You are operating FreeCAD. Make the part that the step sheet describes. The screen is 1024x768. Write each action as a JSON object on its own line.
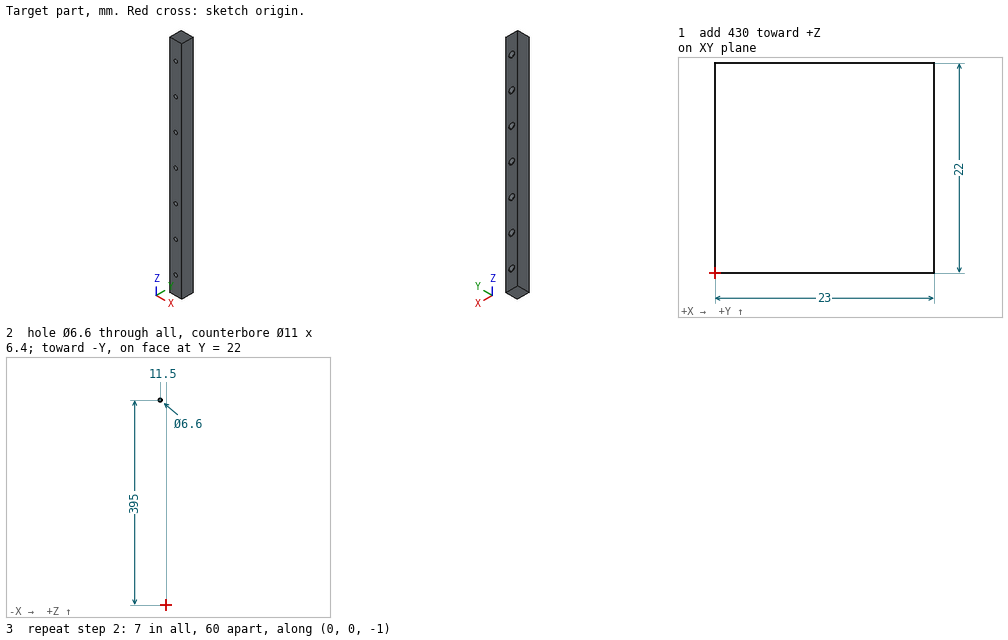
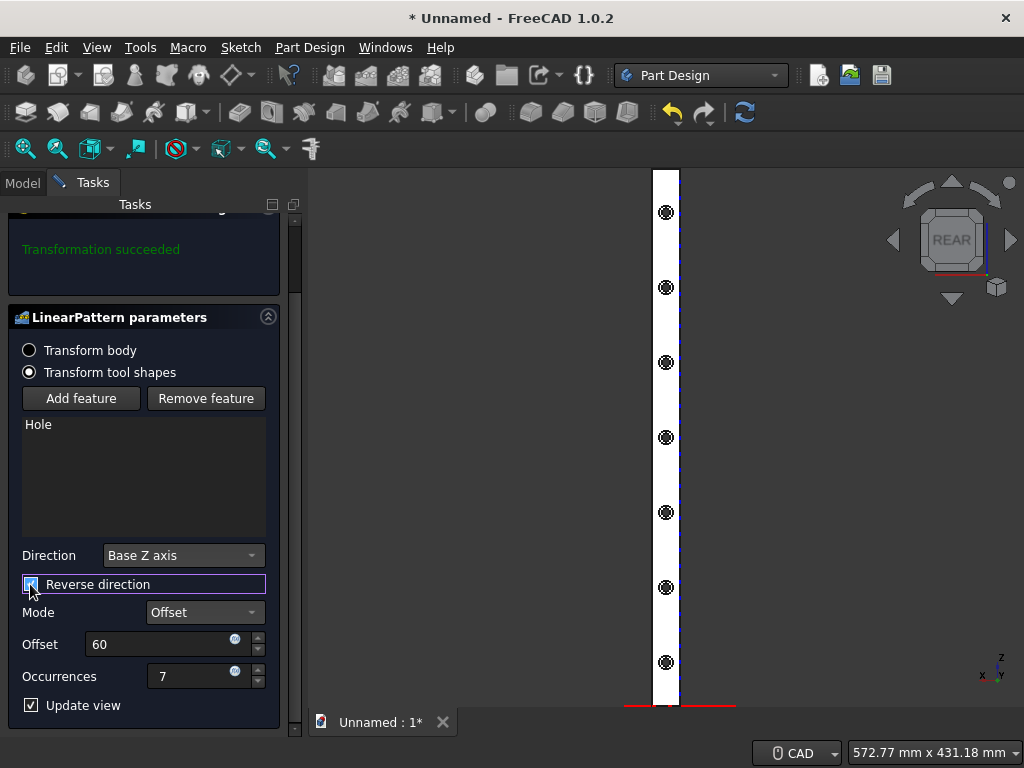
{"action": "scroll", "coordinate": [295, 475], "scroll_direction": "up", "scroll_amount": 3}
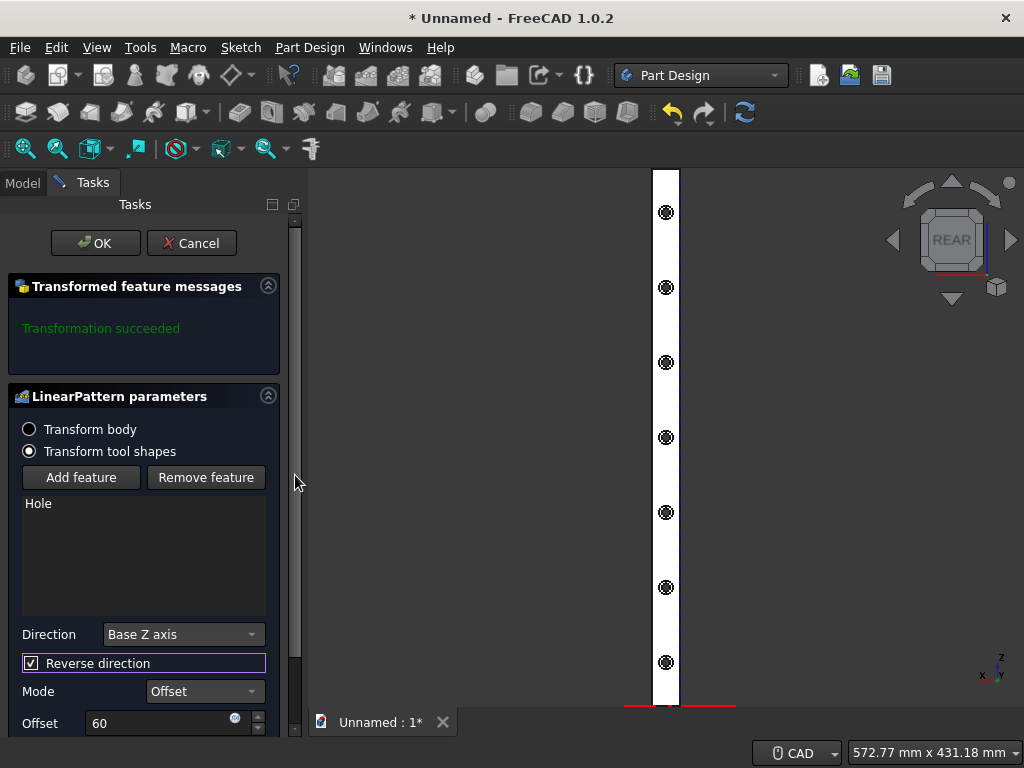
{"action": "left_click", "coordinate": [96, 243]}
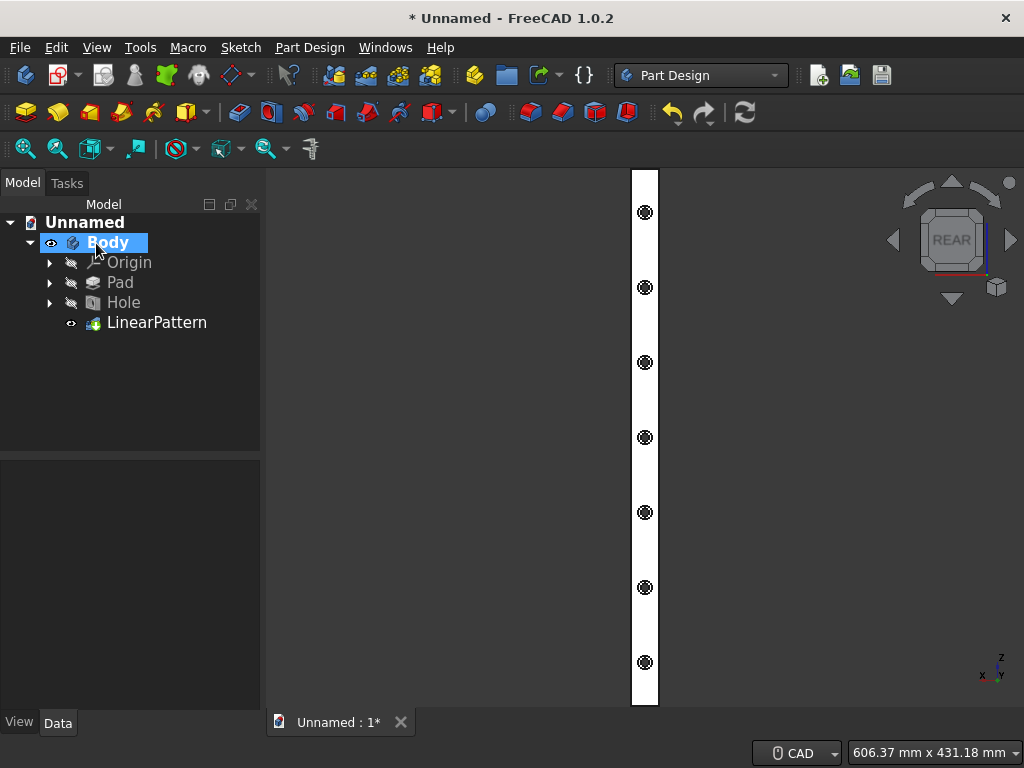
{"action": "key", "text": "0"}